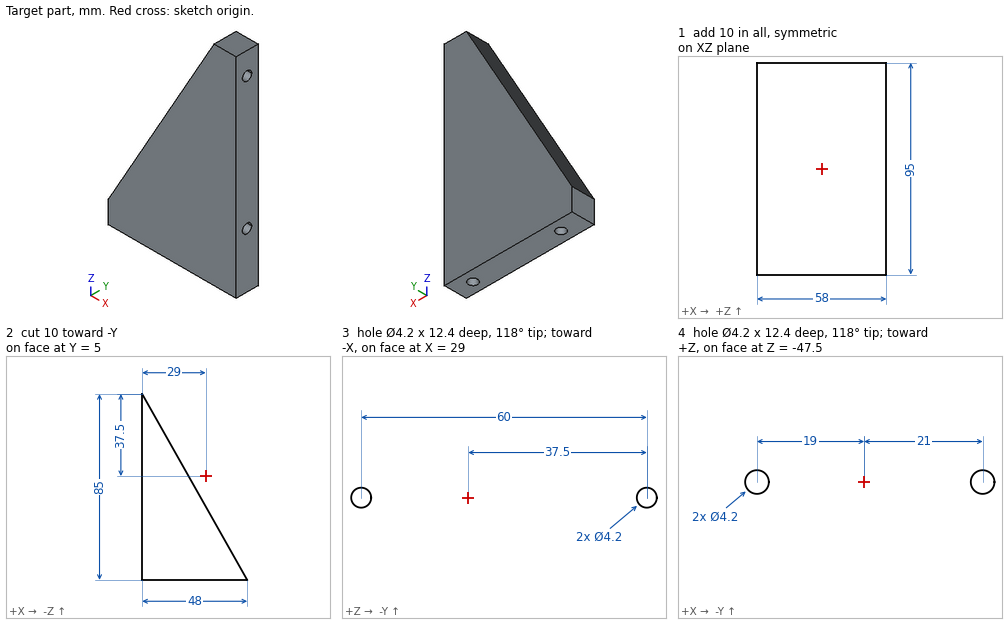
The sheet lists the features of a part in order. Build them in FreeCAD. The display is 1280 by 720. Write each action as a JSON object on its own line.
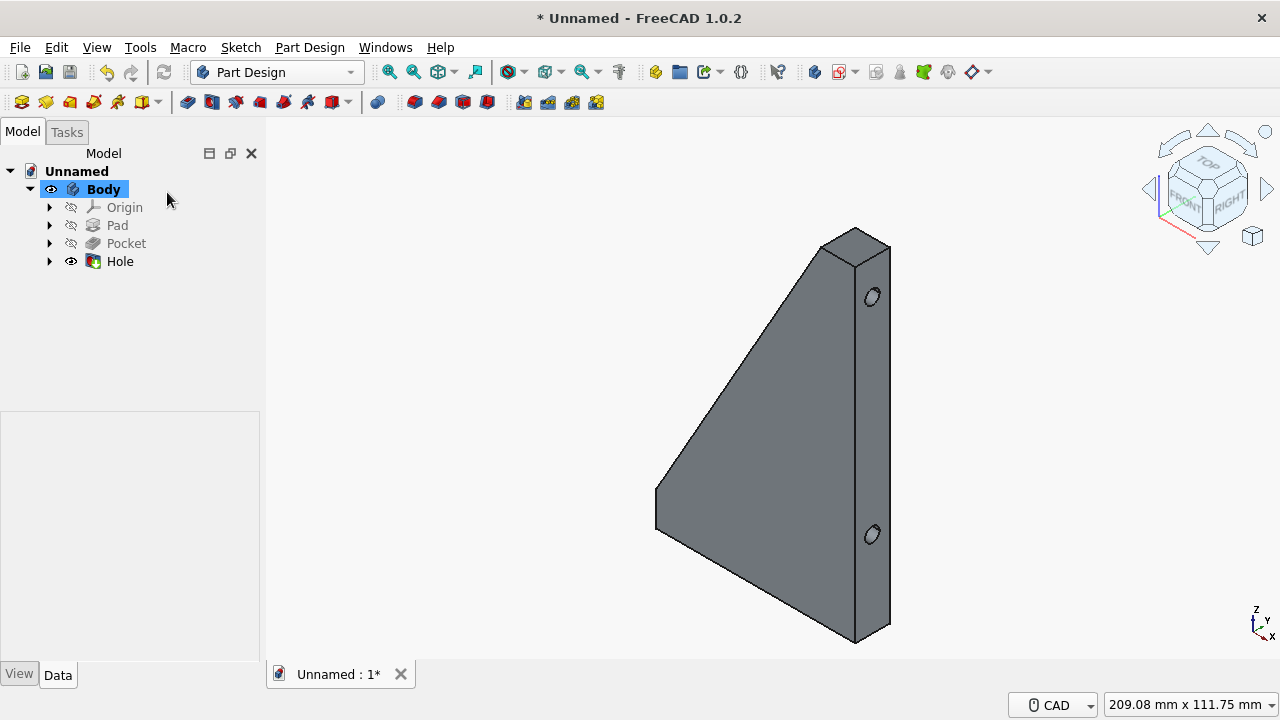
{"action": "key", "text": "5"}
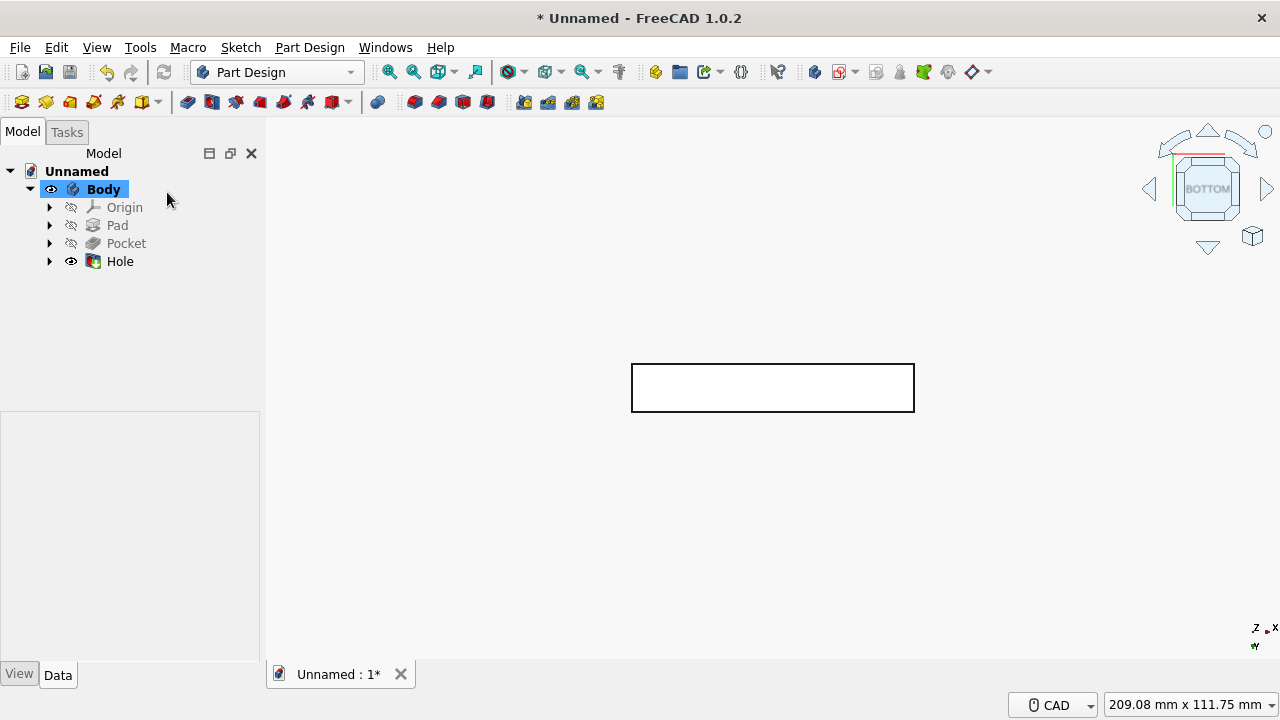
{"action": "left_click", "coordinate": [390, 72]}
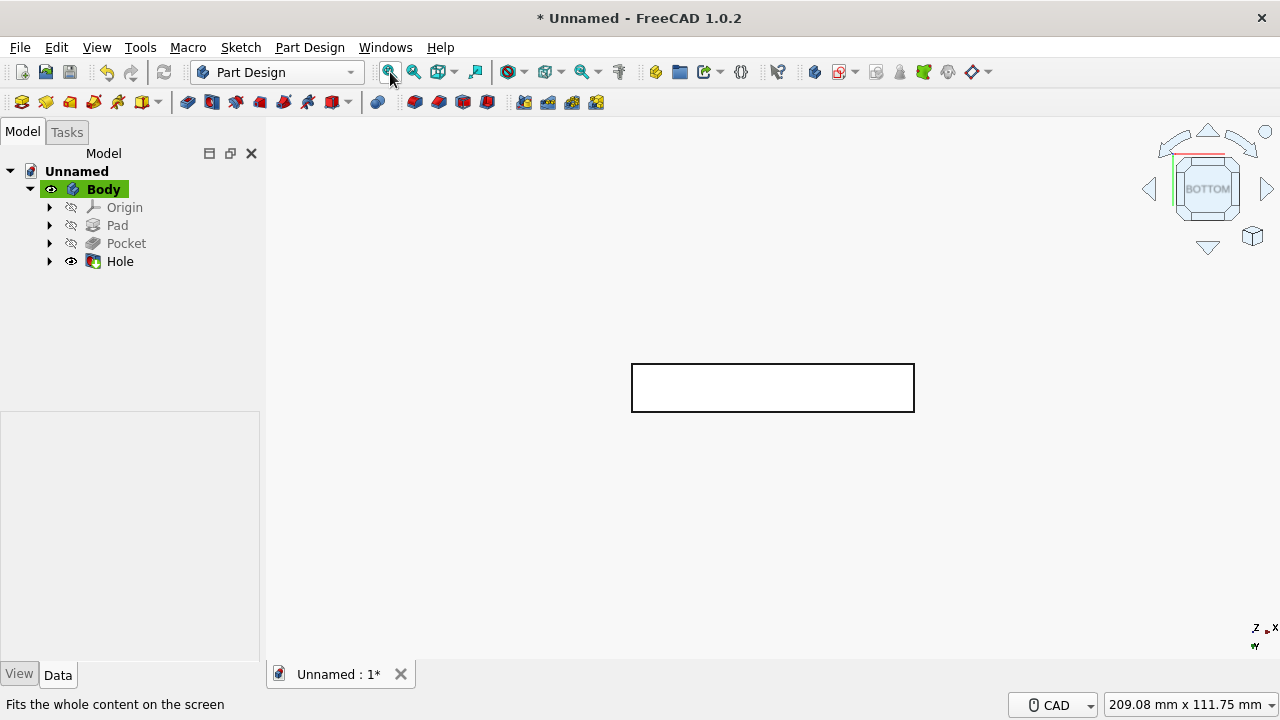
{"action": "left_click", "coordinate": [853, 387]}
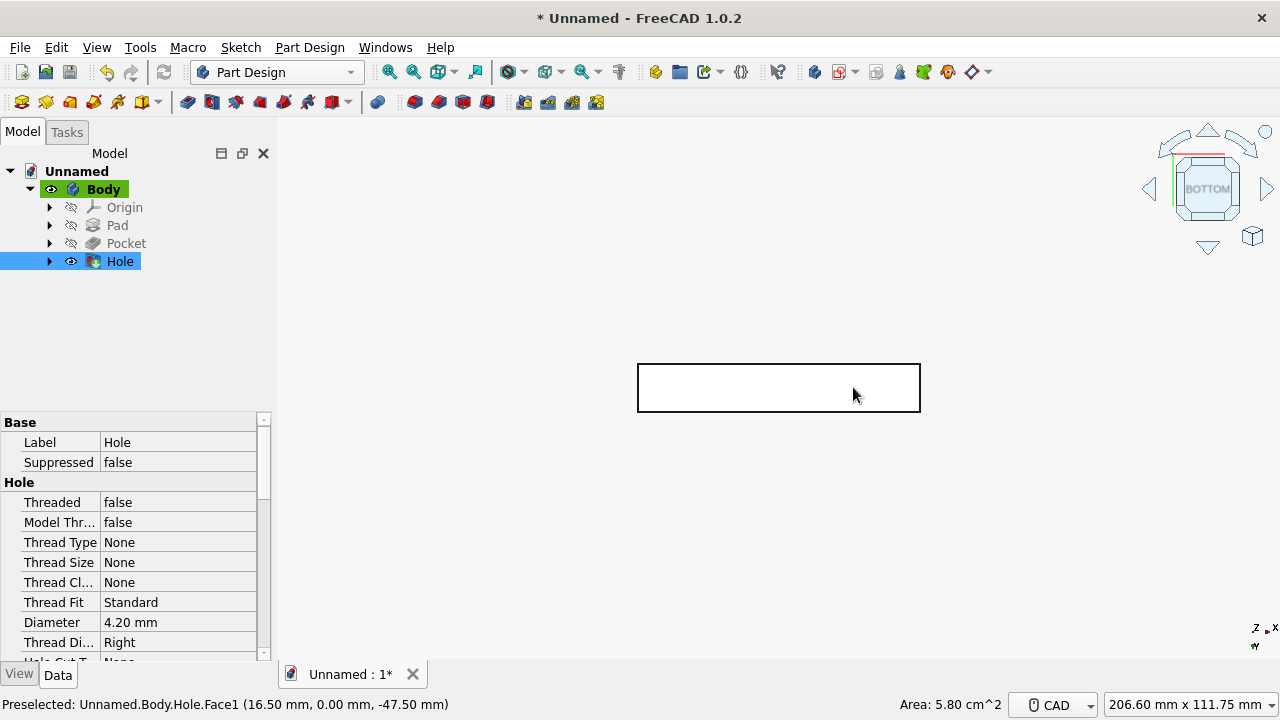
{"action": "left_click", "coordinate": [840, 72]}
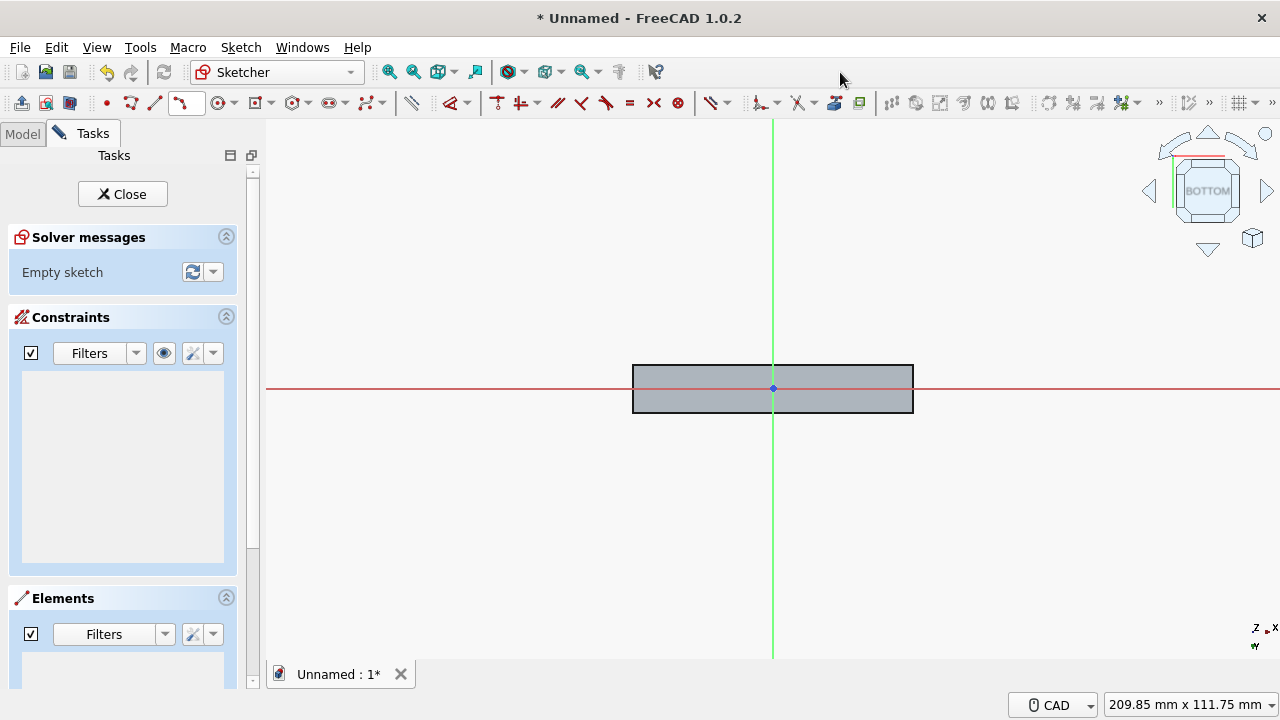
{"action": "scroll", "coordinate": [821, 389], "scroll_direction": "up", "scroll_amount": 5}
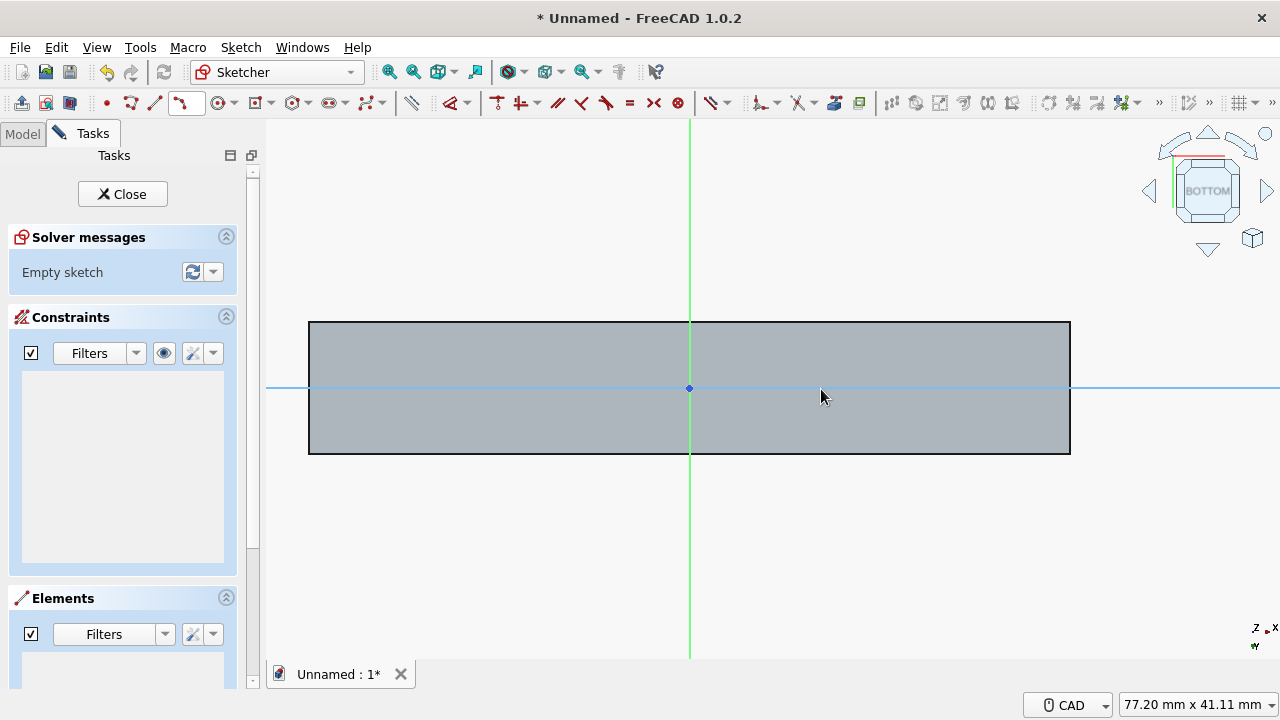
{"action": "left_click", "coordinate": [218, 104]}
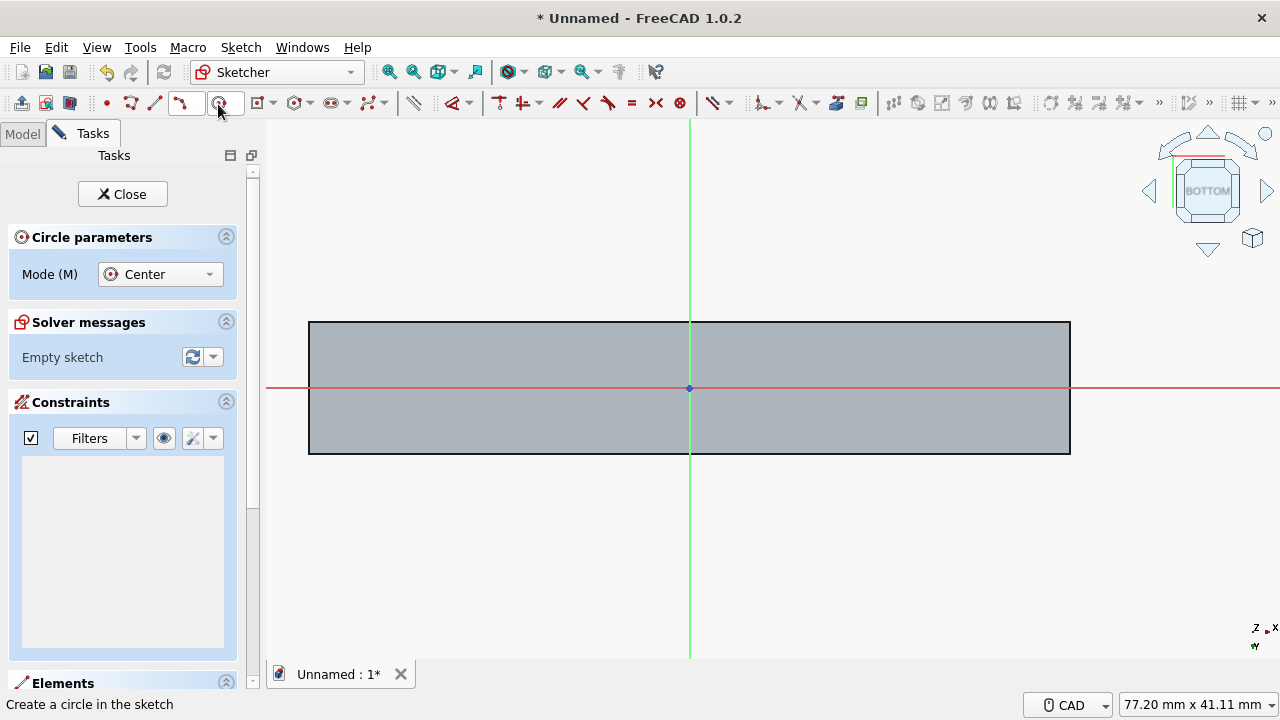
{"action": "left_click", "coordinate": [440, 388]}
{"action": "left_click", "coordinate": [460, 369]}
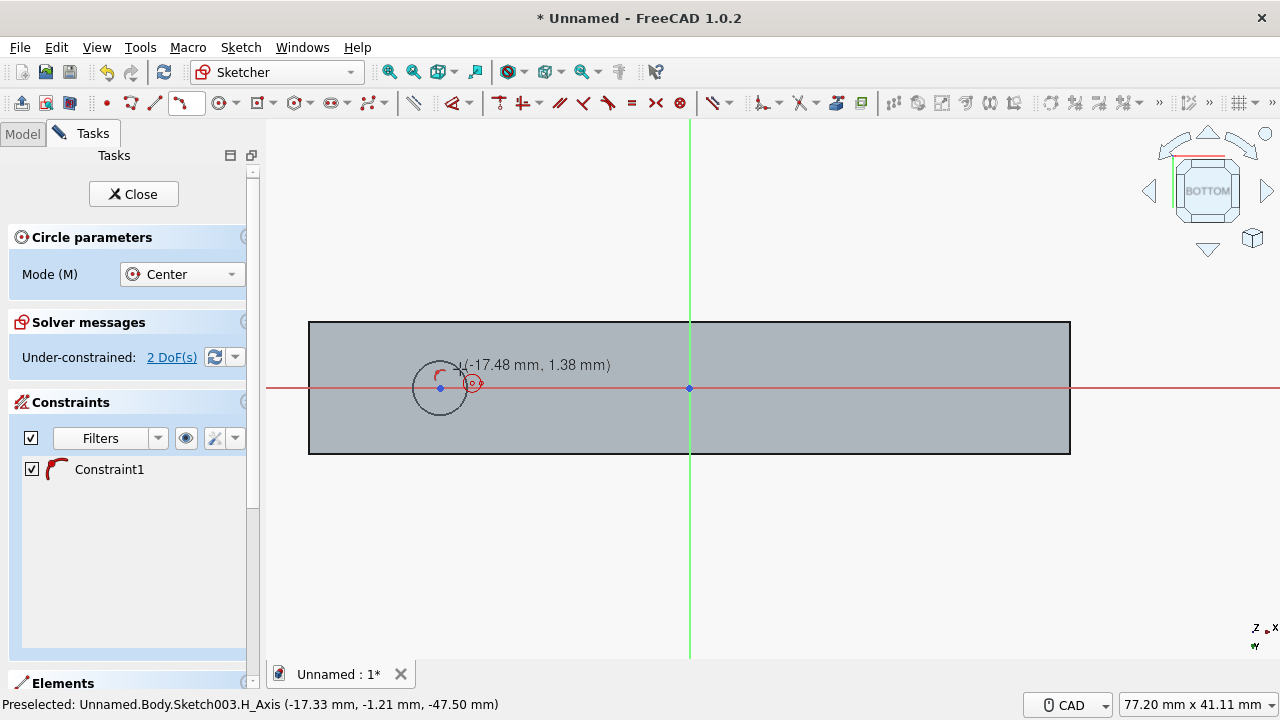
{"action": "left_click", "coordinate": [965, 388]}
{"action": "left_click", "coordinate": [985, 369]}
{"action": "key", "text": "Escape"}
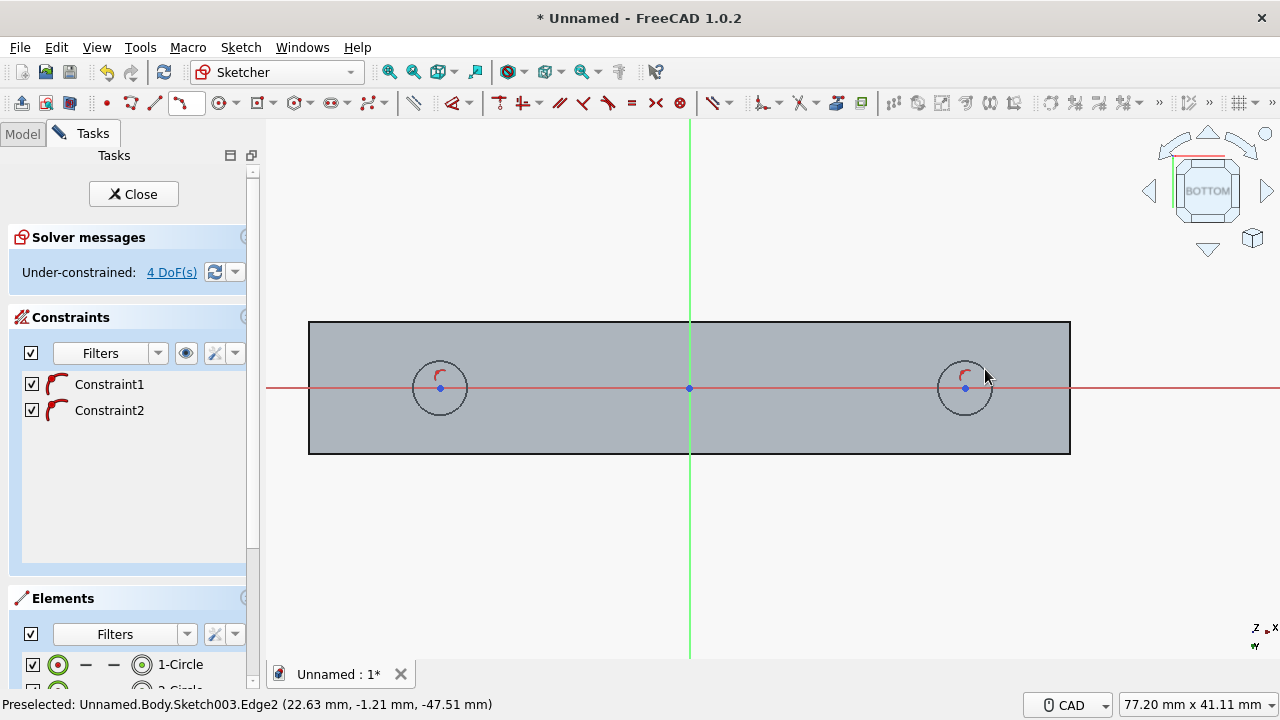
{"action": "left_click", "coordinate": [459, 369]}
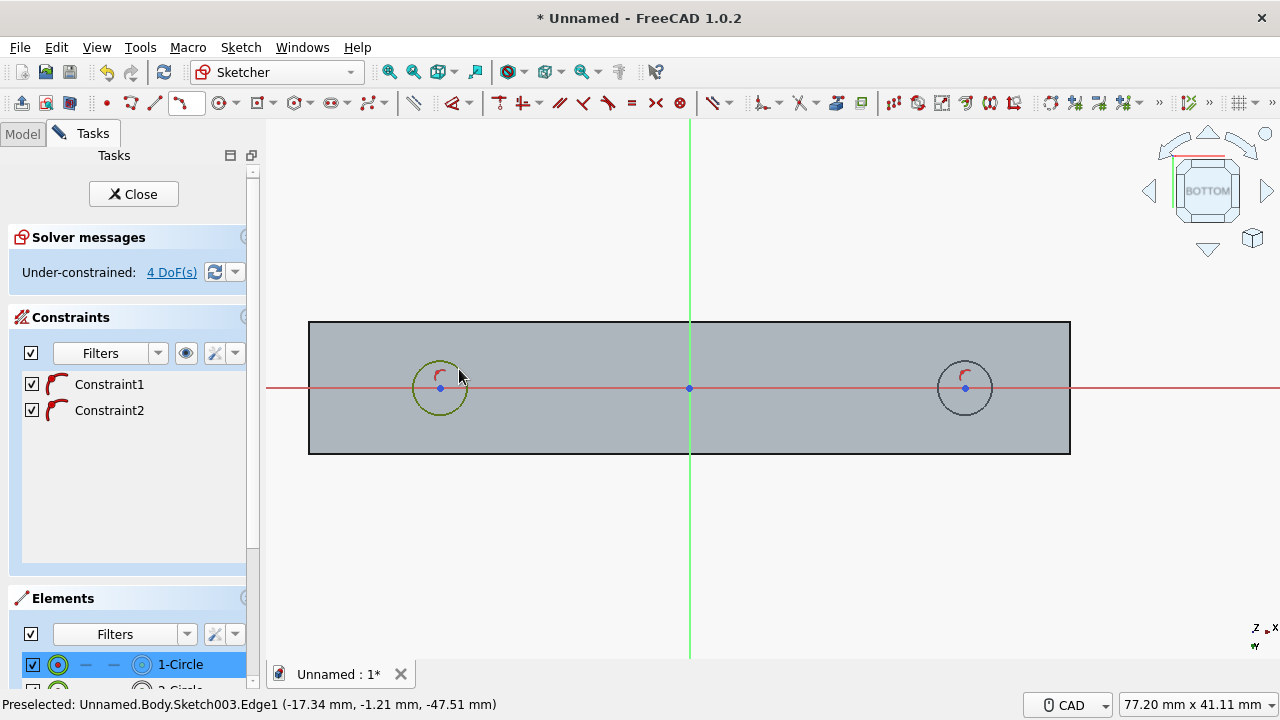
{"action": "left_click", "coordinate": [984, 369]}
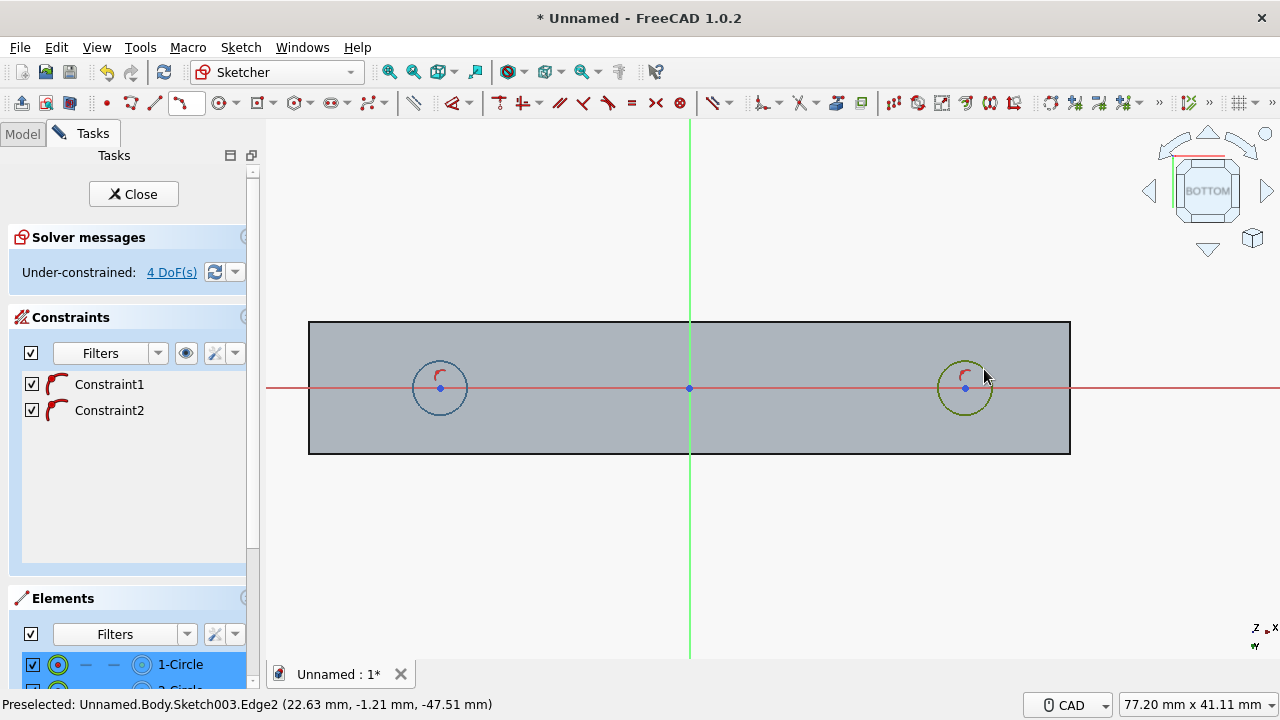
{"action": "left_click", "coordinate": [632, 104]}